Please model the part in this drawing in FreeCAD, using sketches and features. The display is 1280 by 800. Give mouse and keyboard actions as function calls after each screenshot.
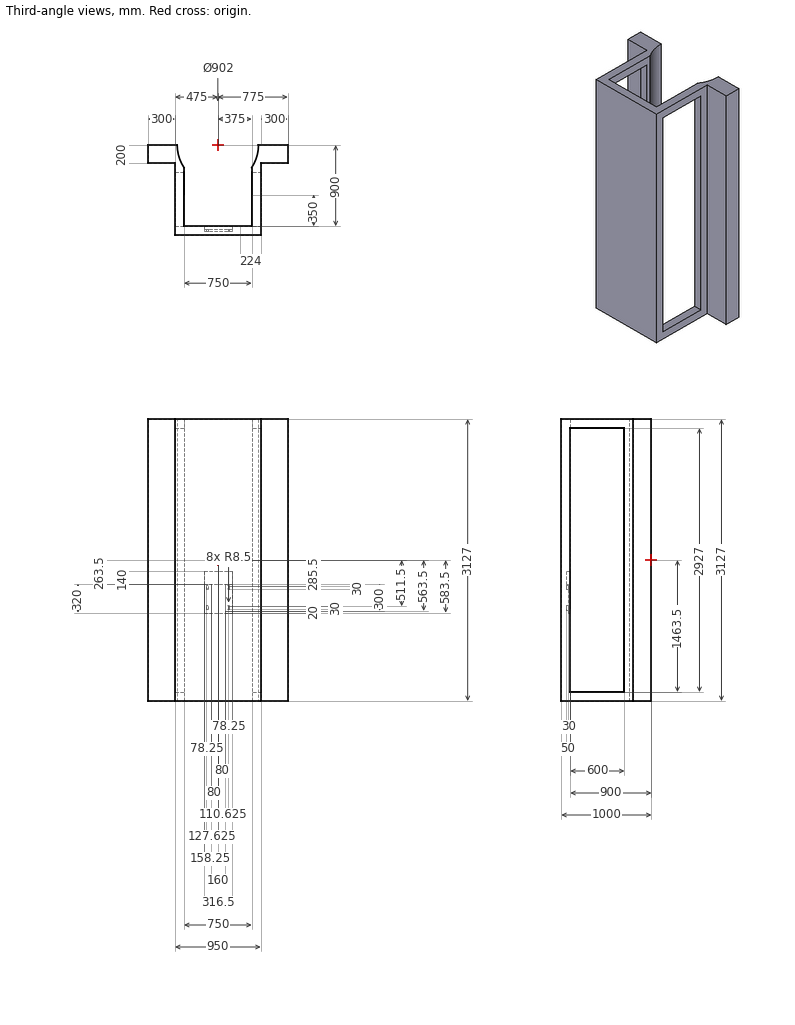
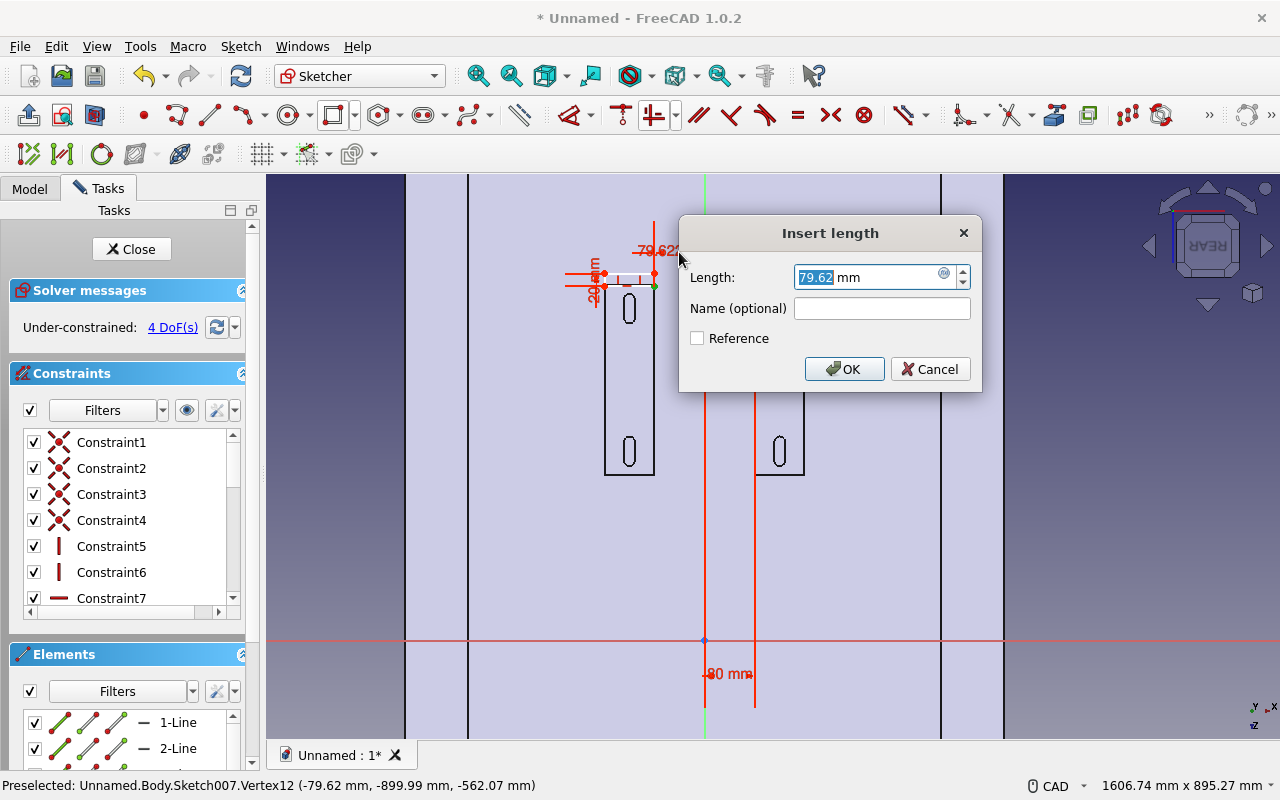
text(80)
key(Return)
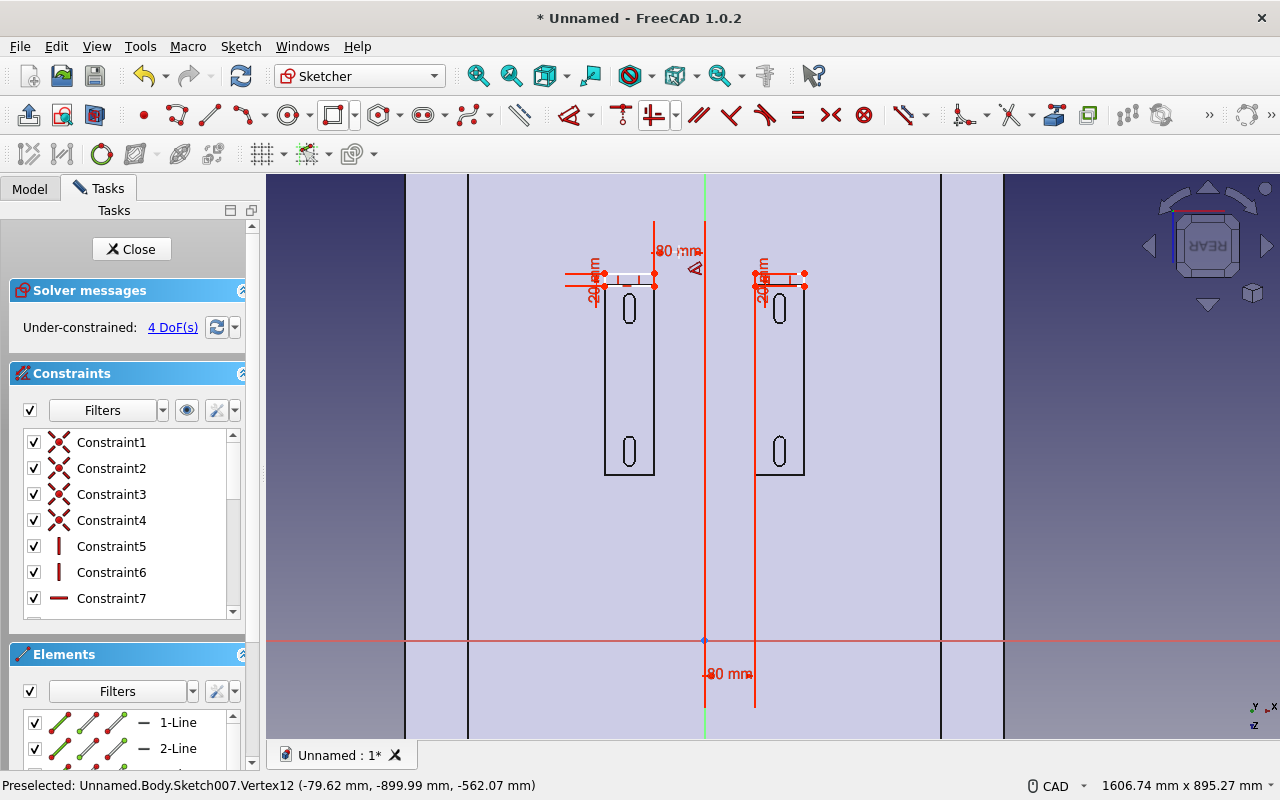
click(770, 286)
click(780, 252)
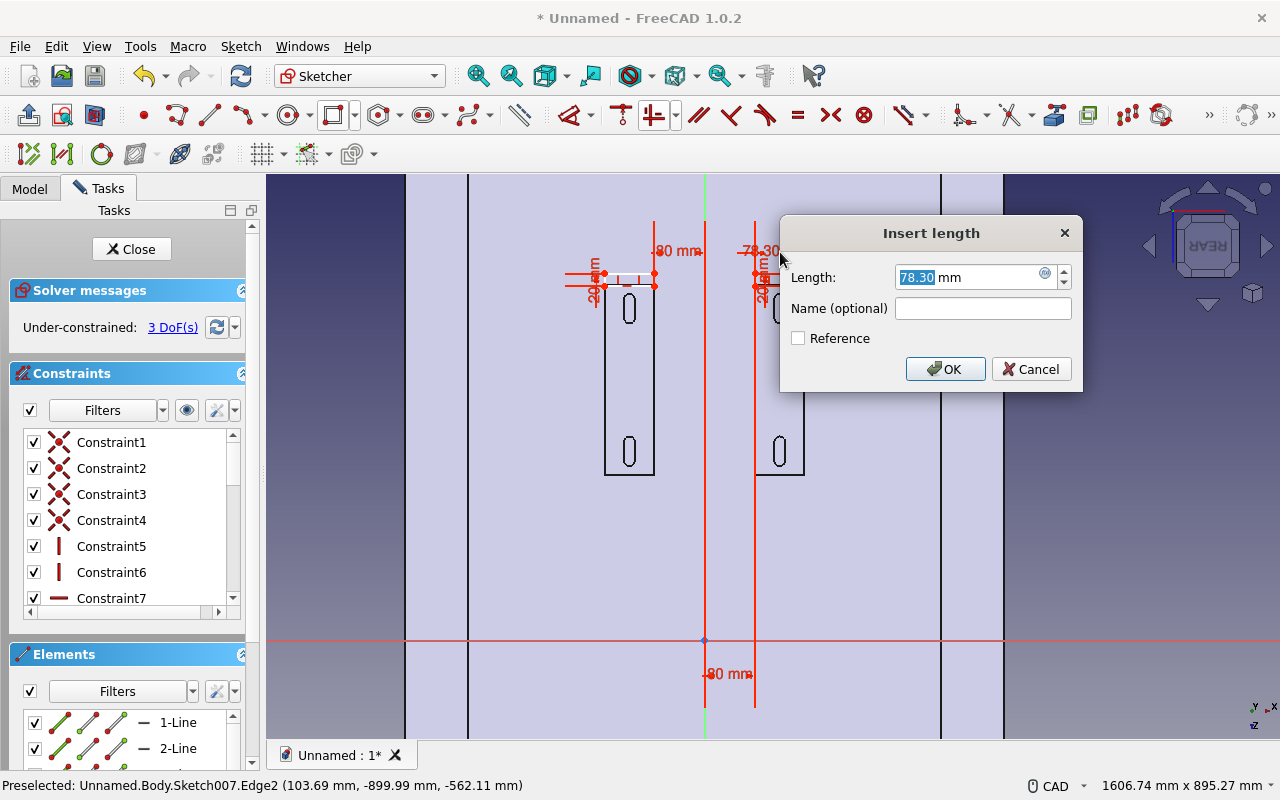
text(78.25)
key(Return)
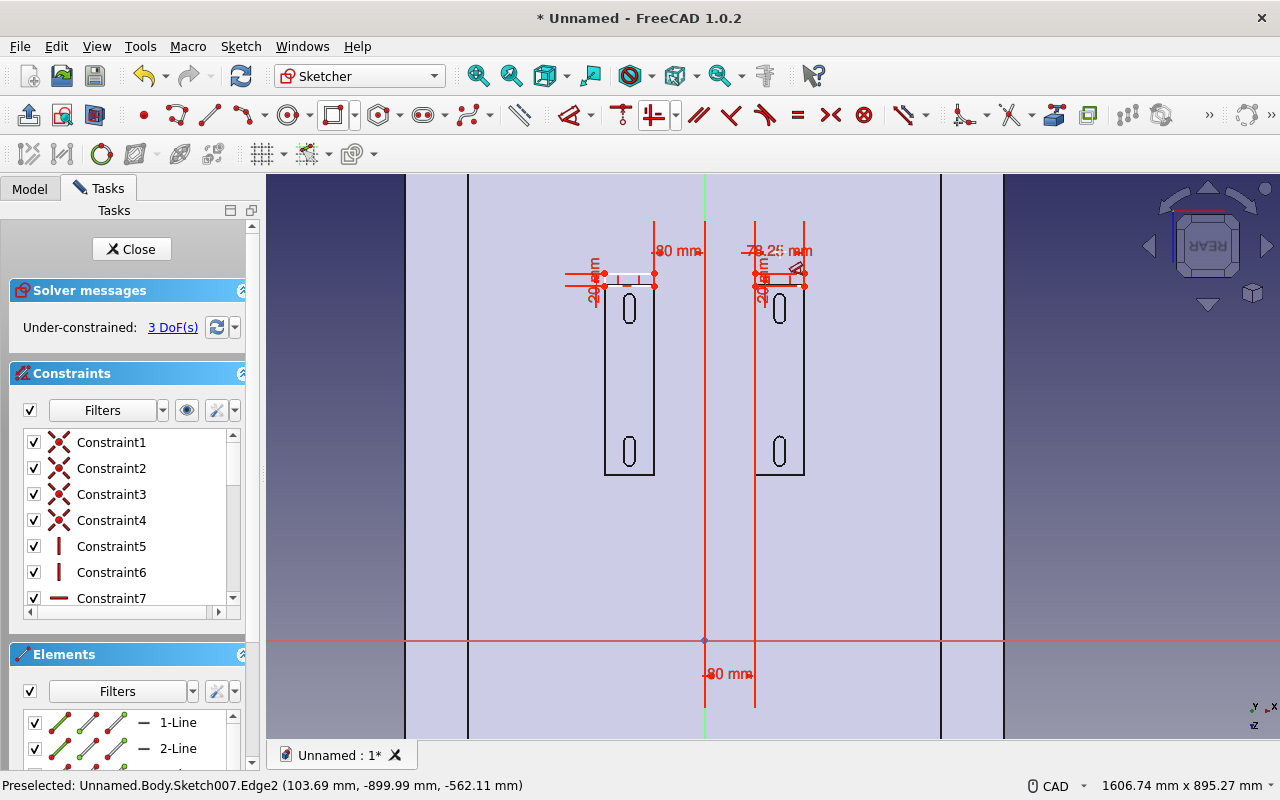
click(620, 286)
click(629, 320)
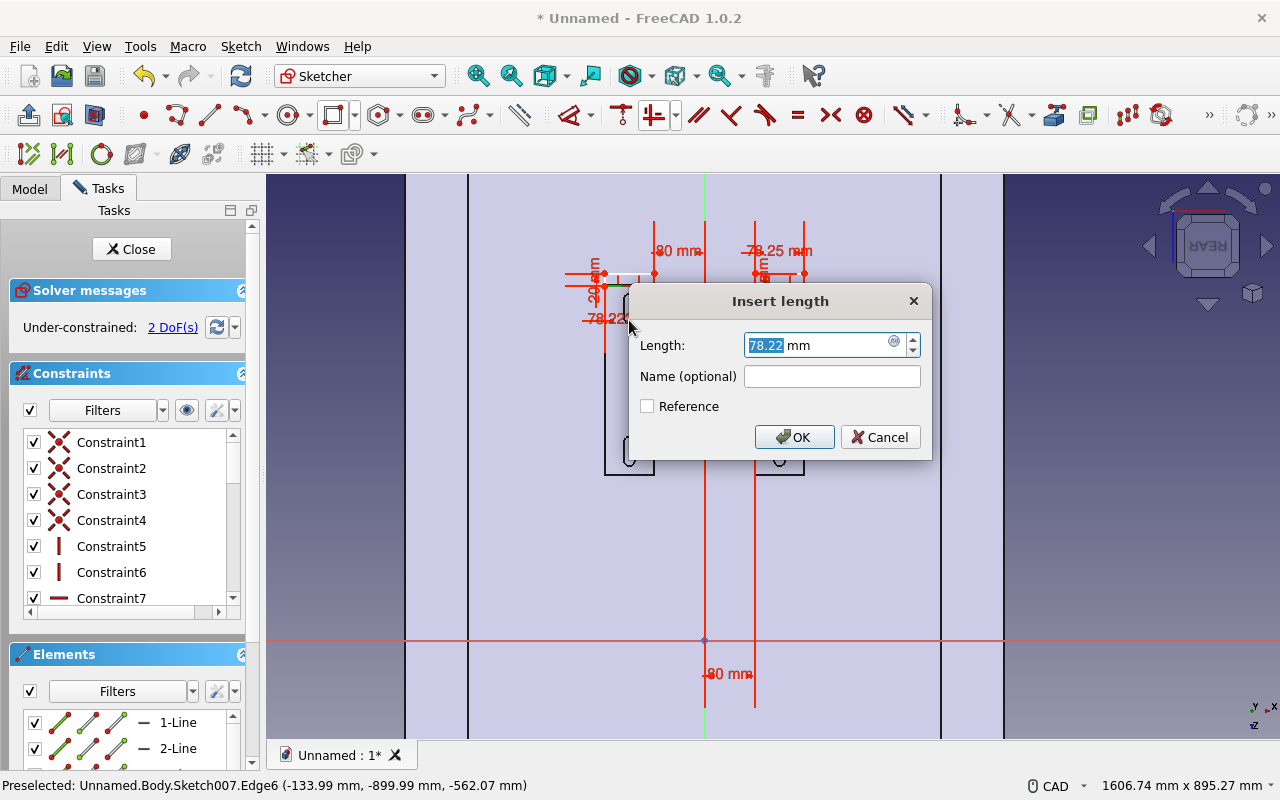
text(78.25)
key(Return)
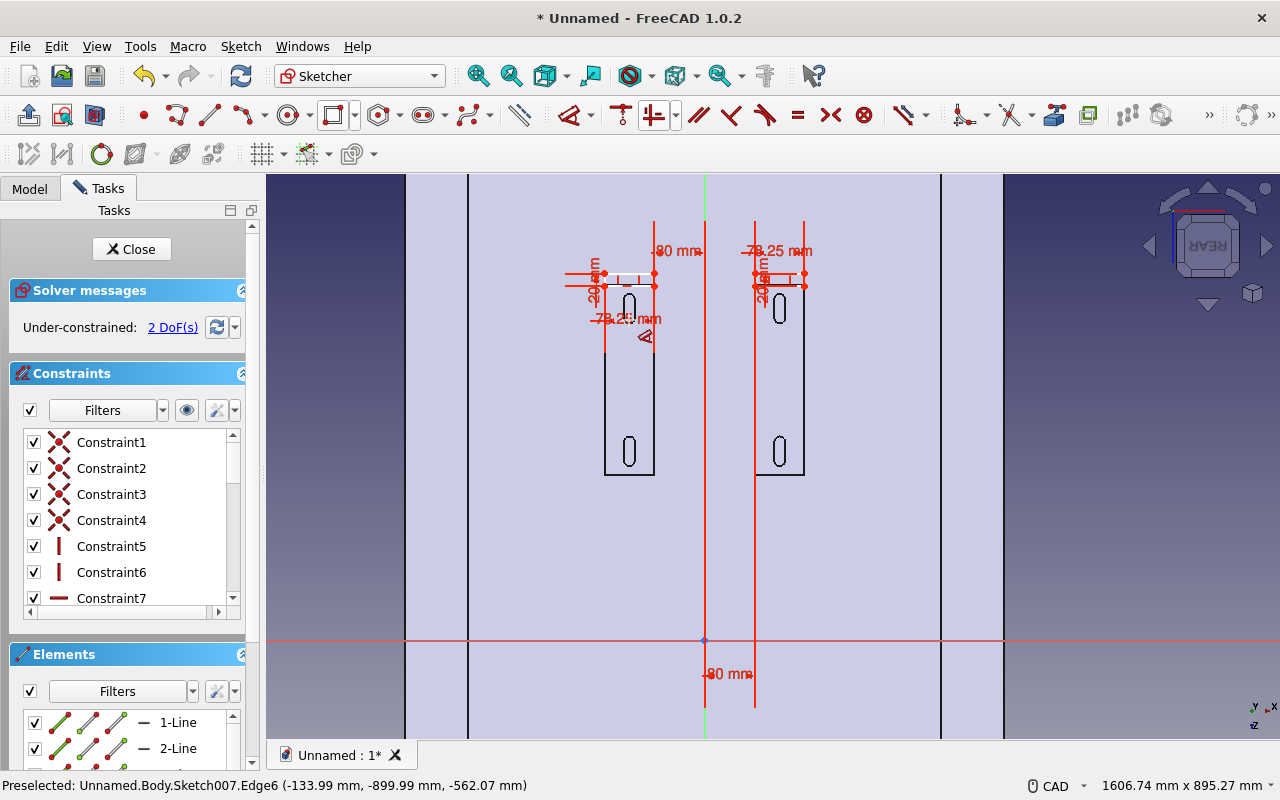
click(755, 274)
click(789, 457)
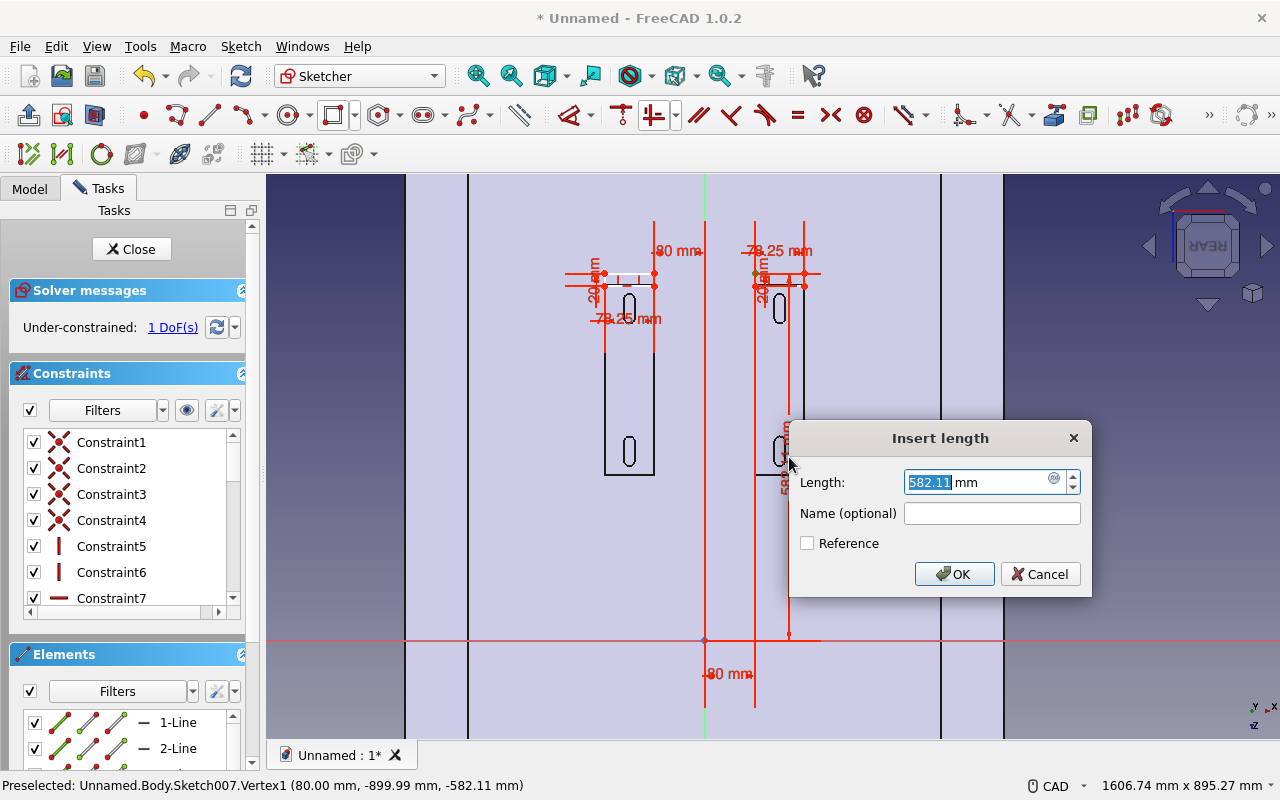
text(583.5)
key(Return)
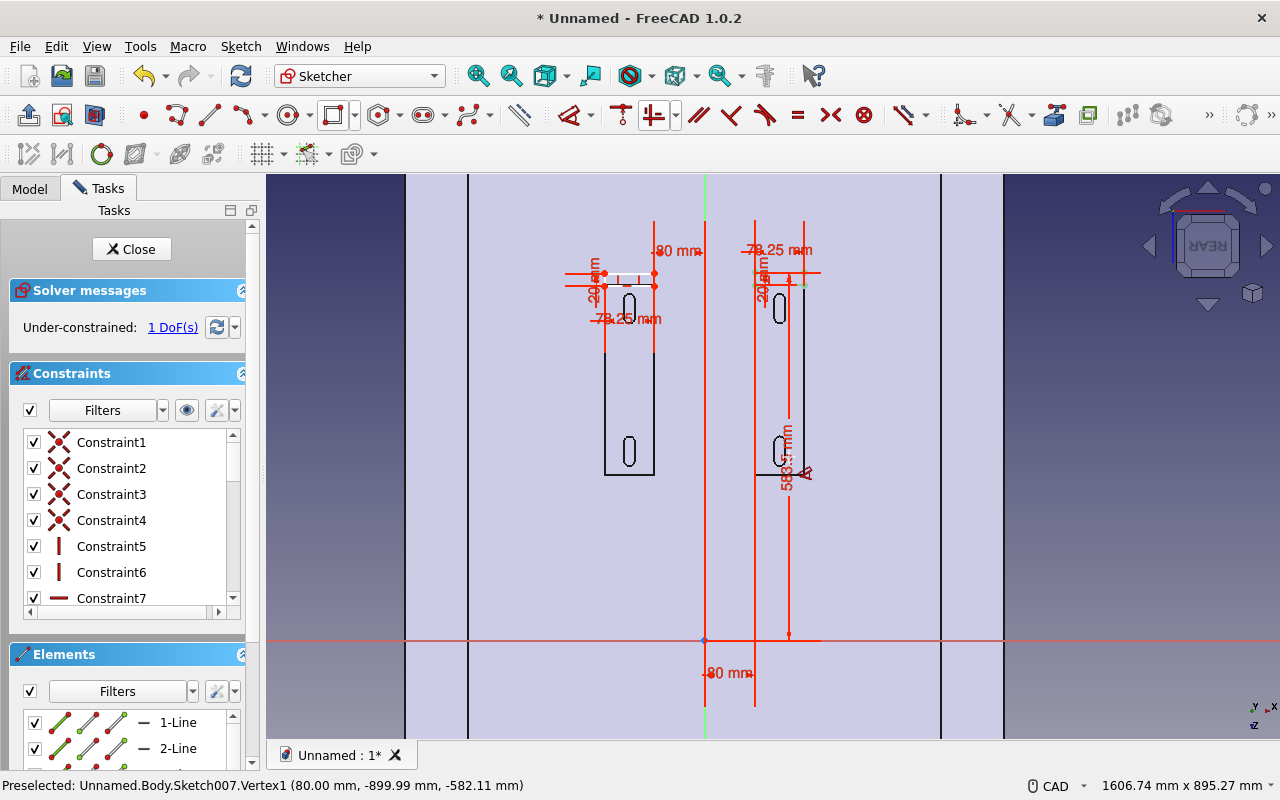
click(605, 274)
click(571, 457)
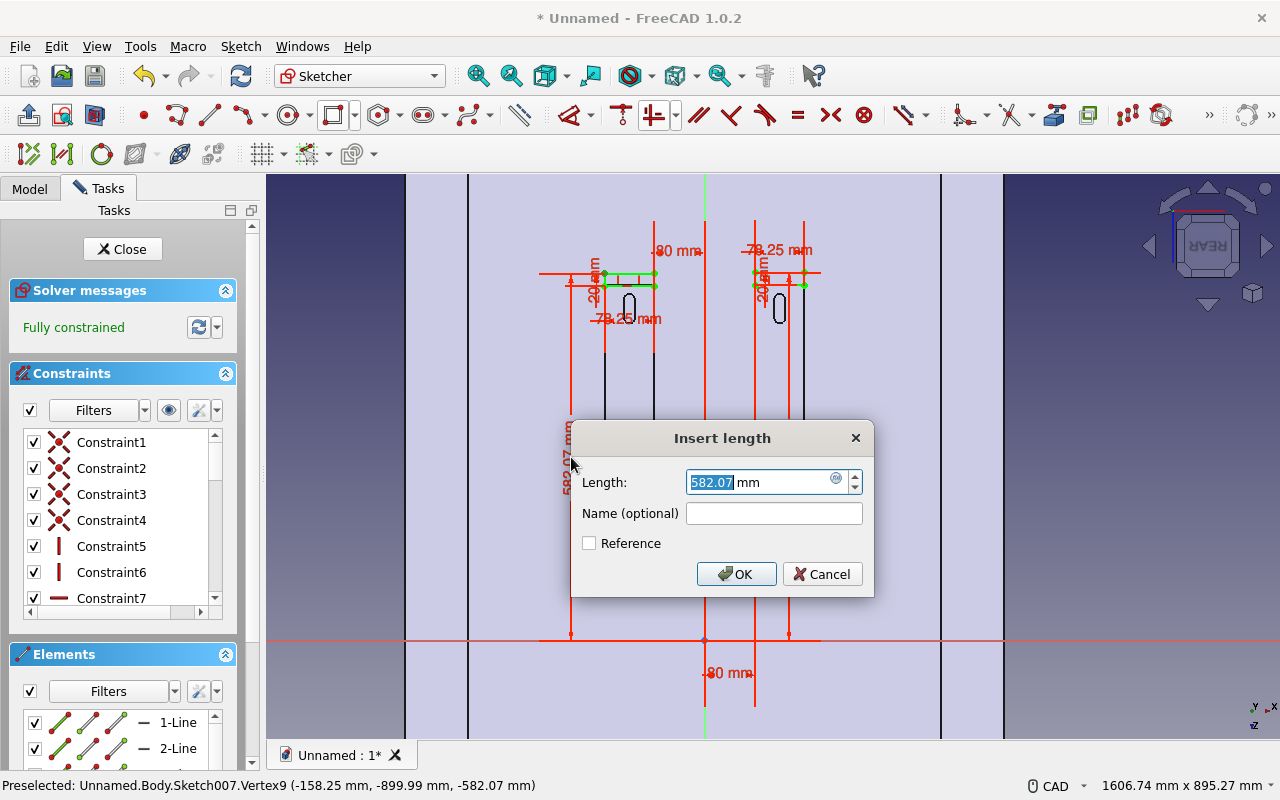
text(583.5)
key(Return)
key(Escape)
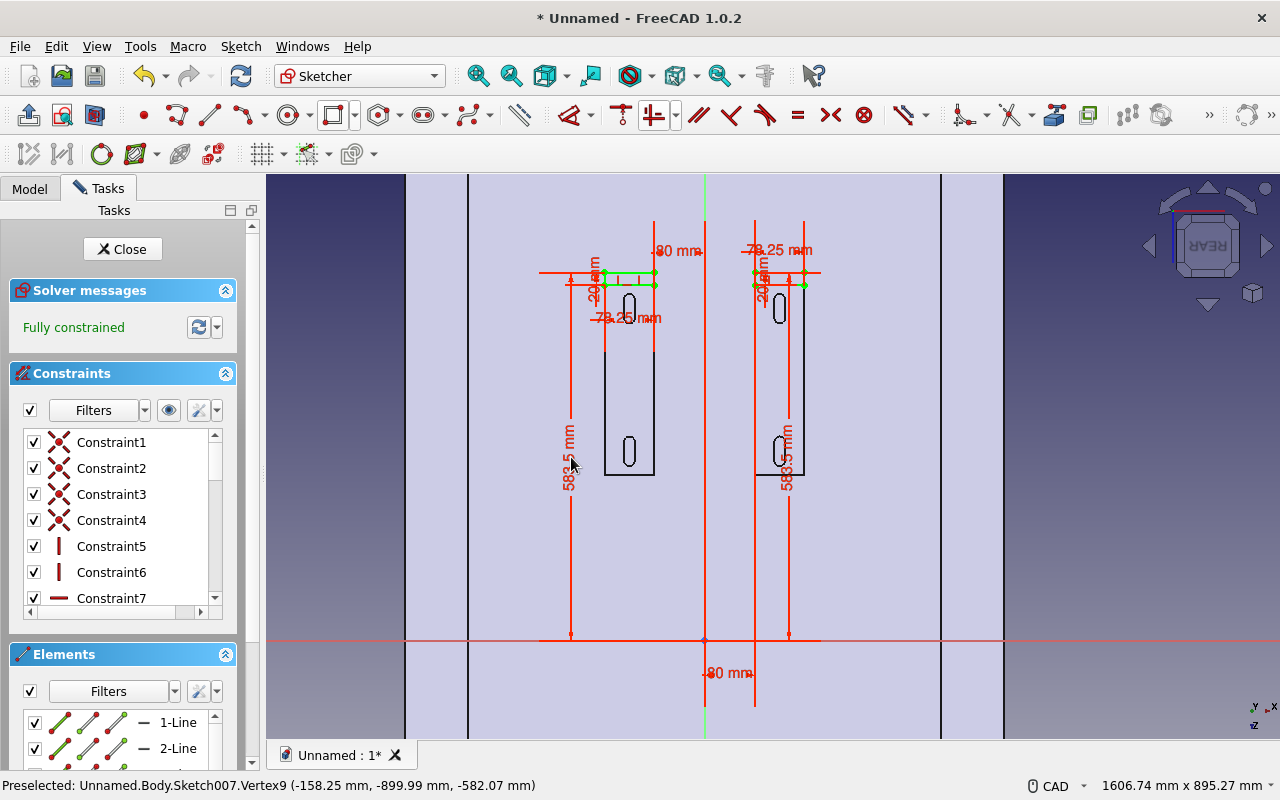
click(123, 249)